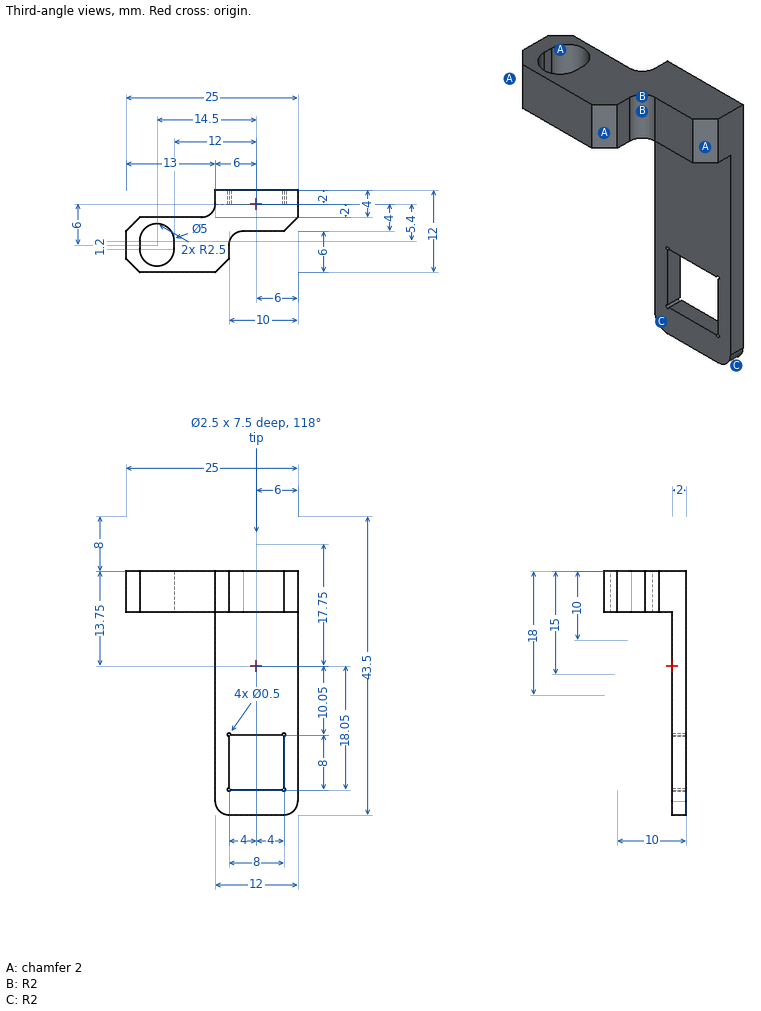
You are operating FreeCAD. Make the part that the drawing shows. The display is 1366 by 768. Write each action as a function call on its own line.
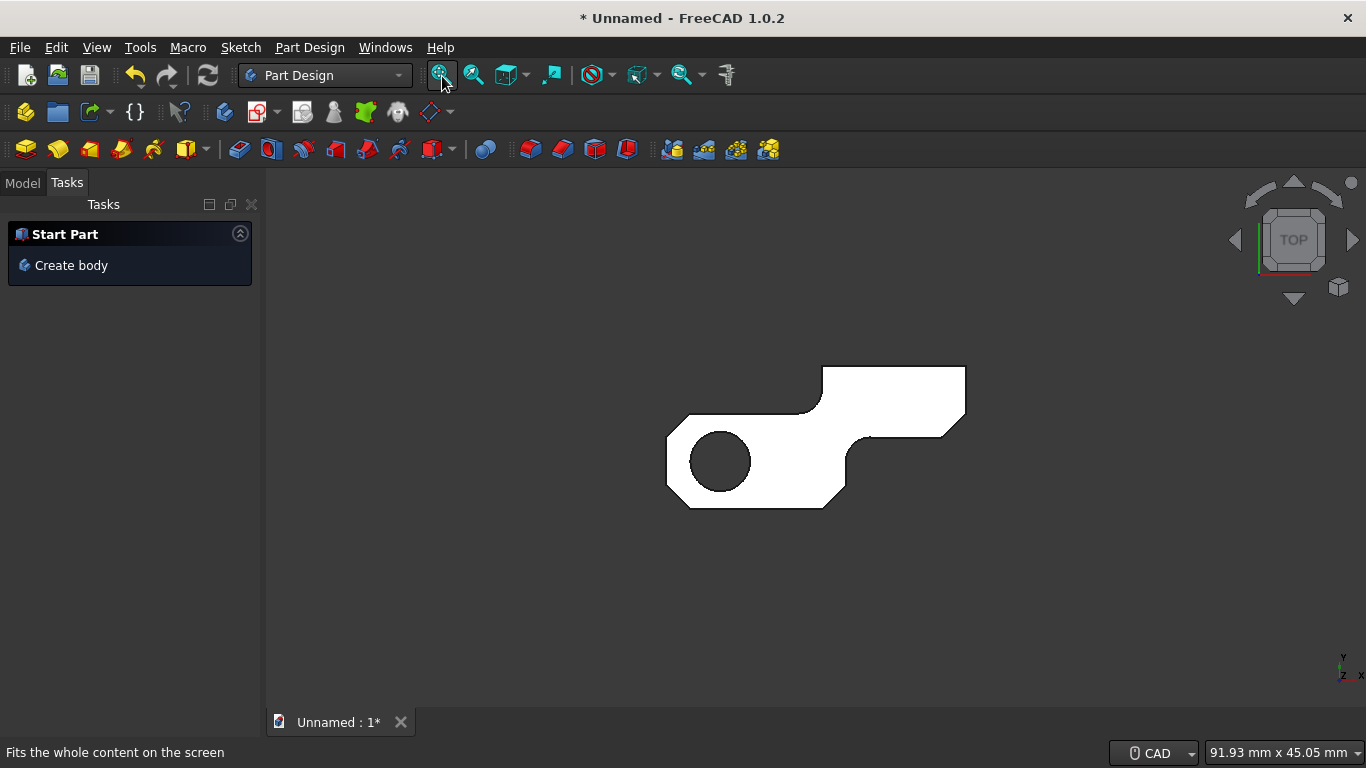
key(0)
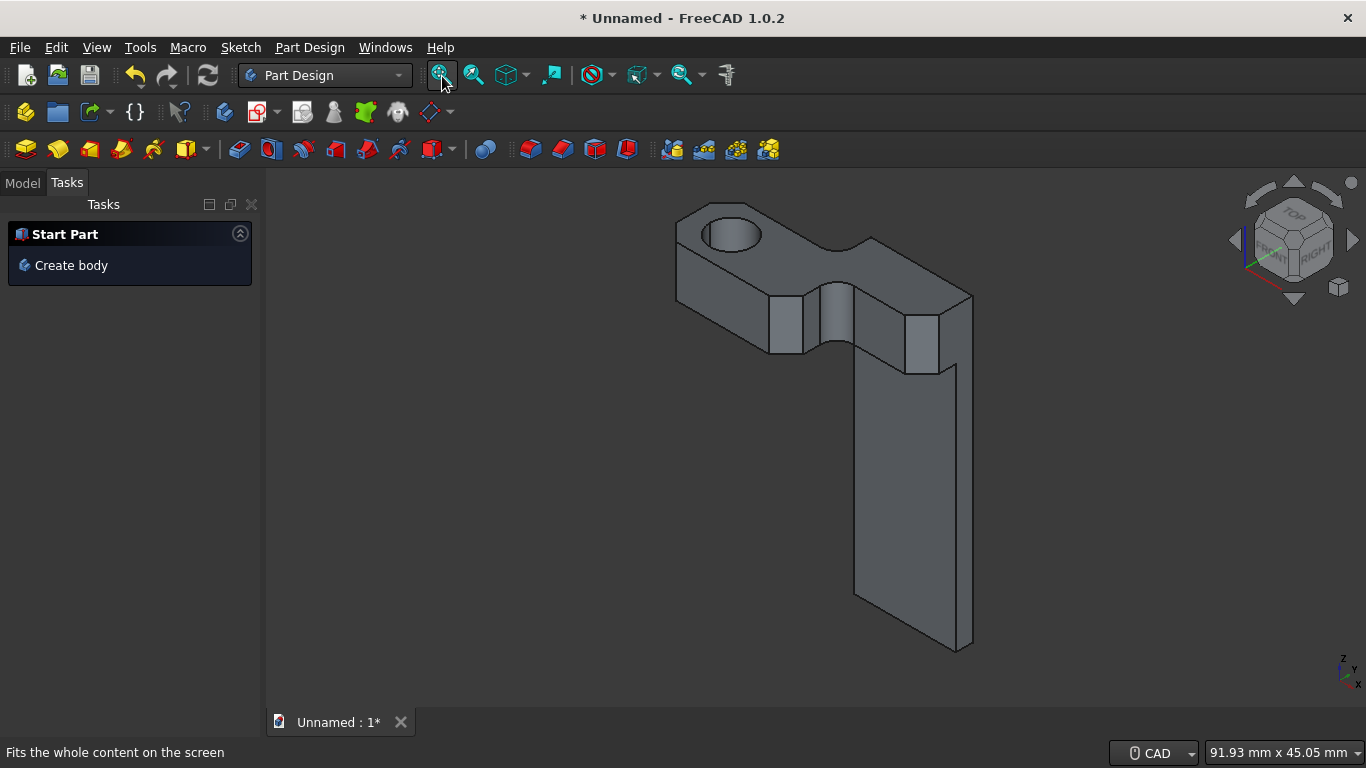
key(1)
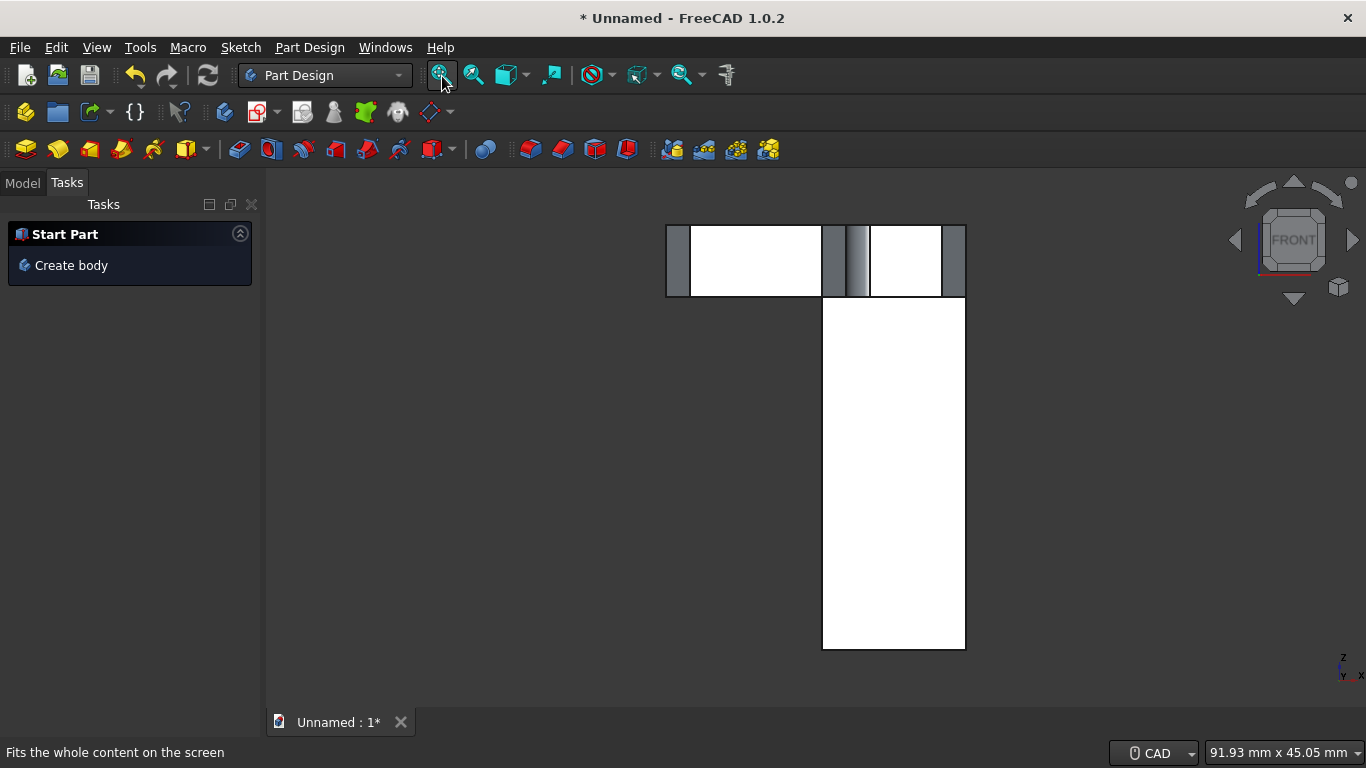
key(3)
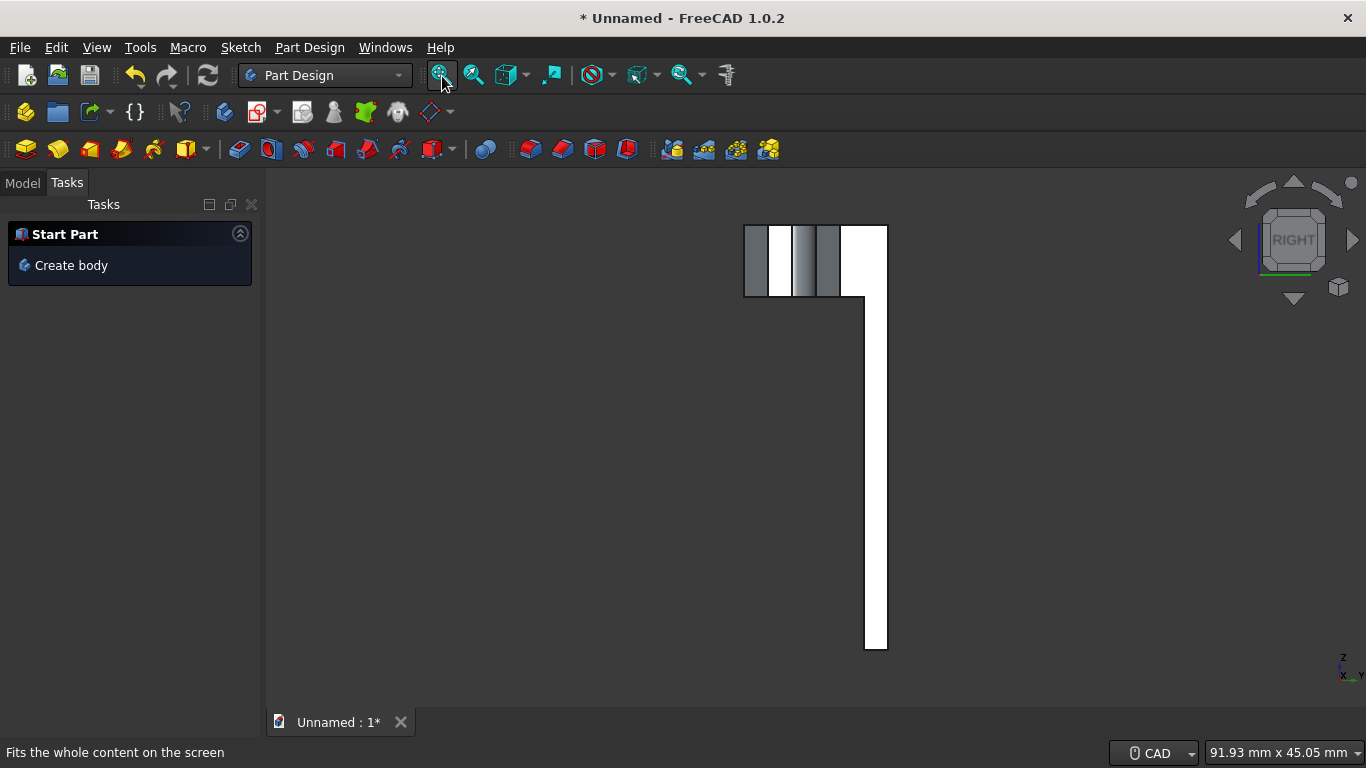
click(876, 649)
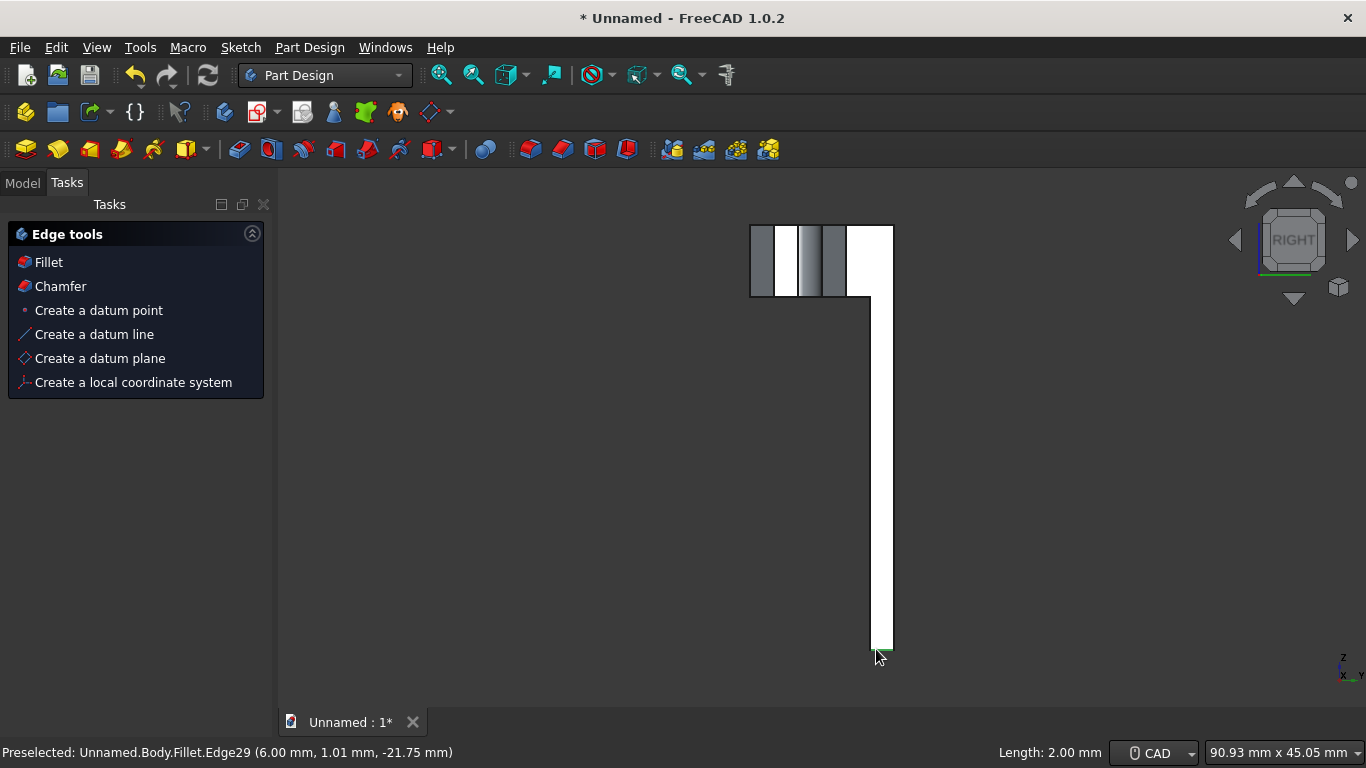
key(5)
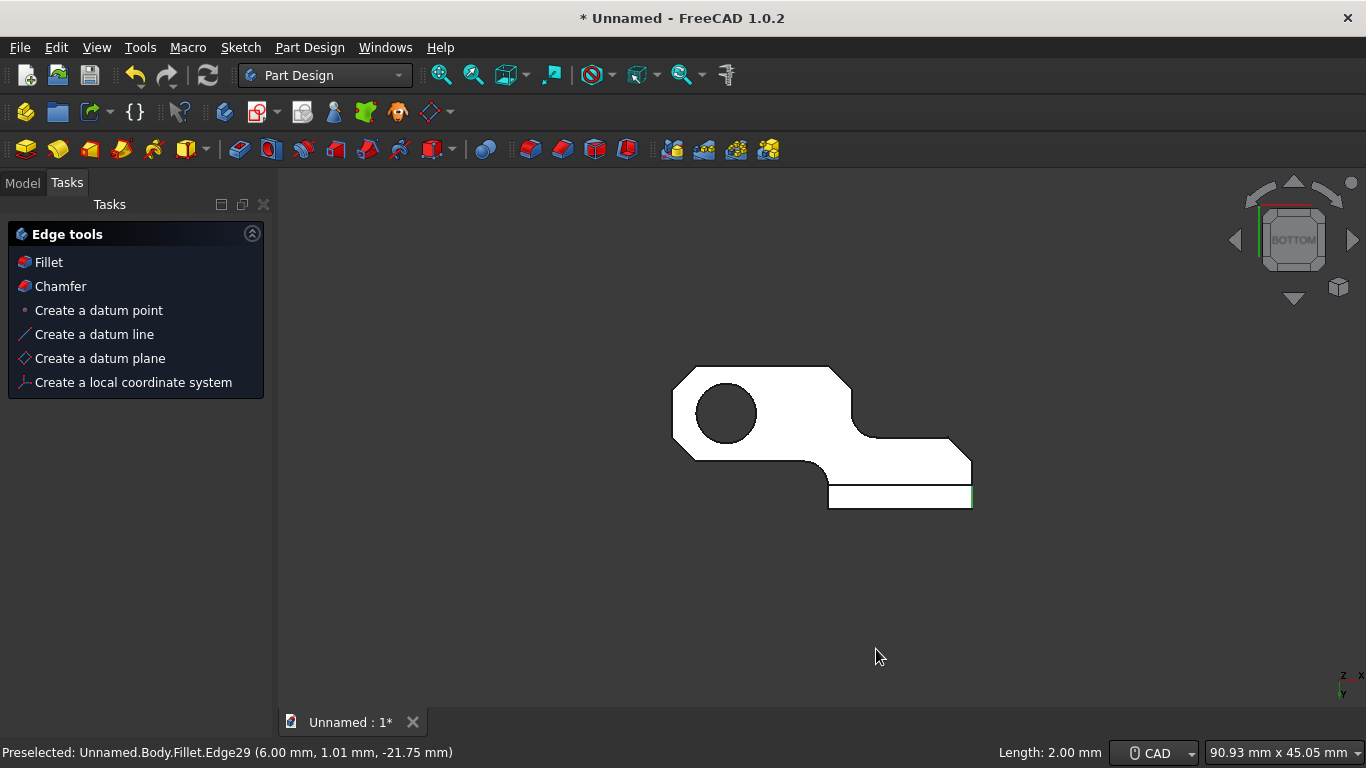
click(442, 76)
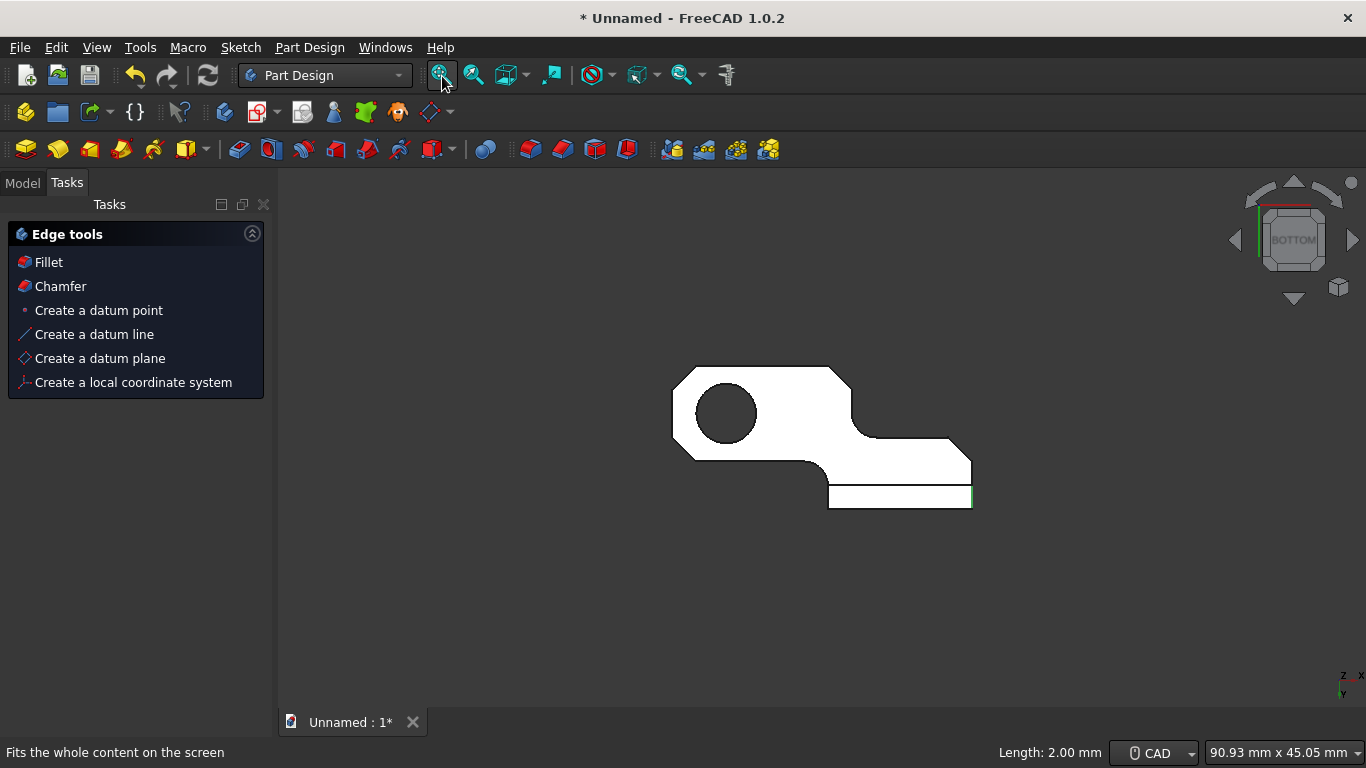
click(828, 496, ctrl)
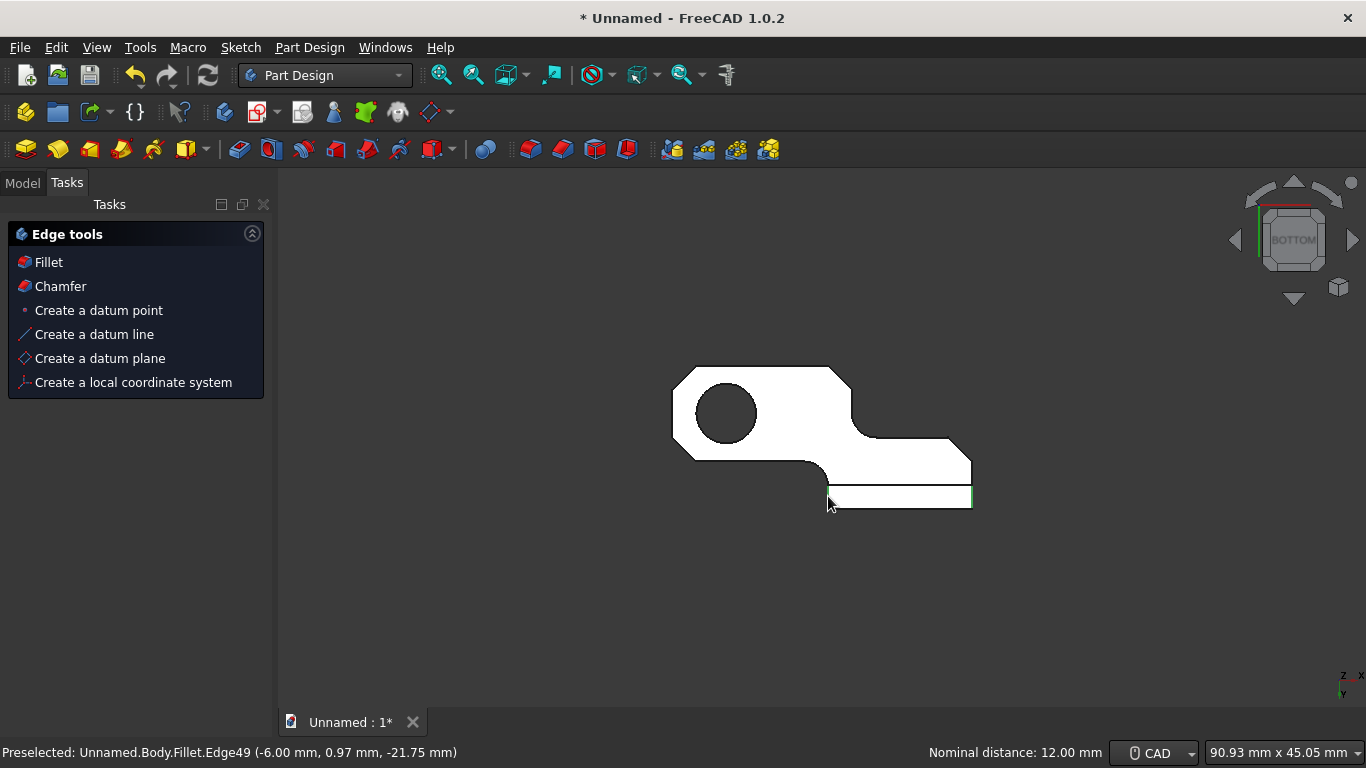
click(532, 150)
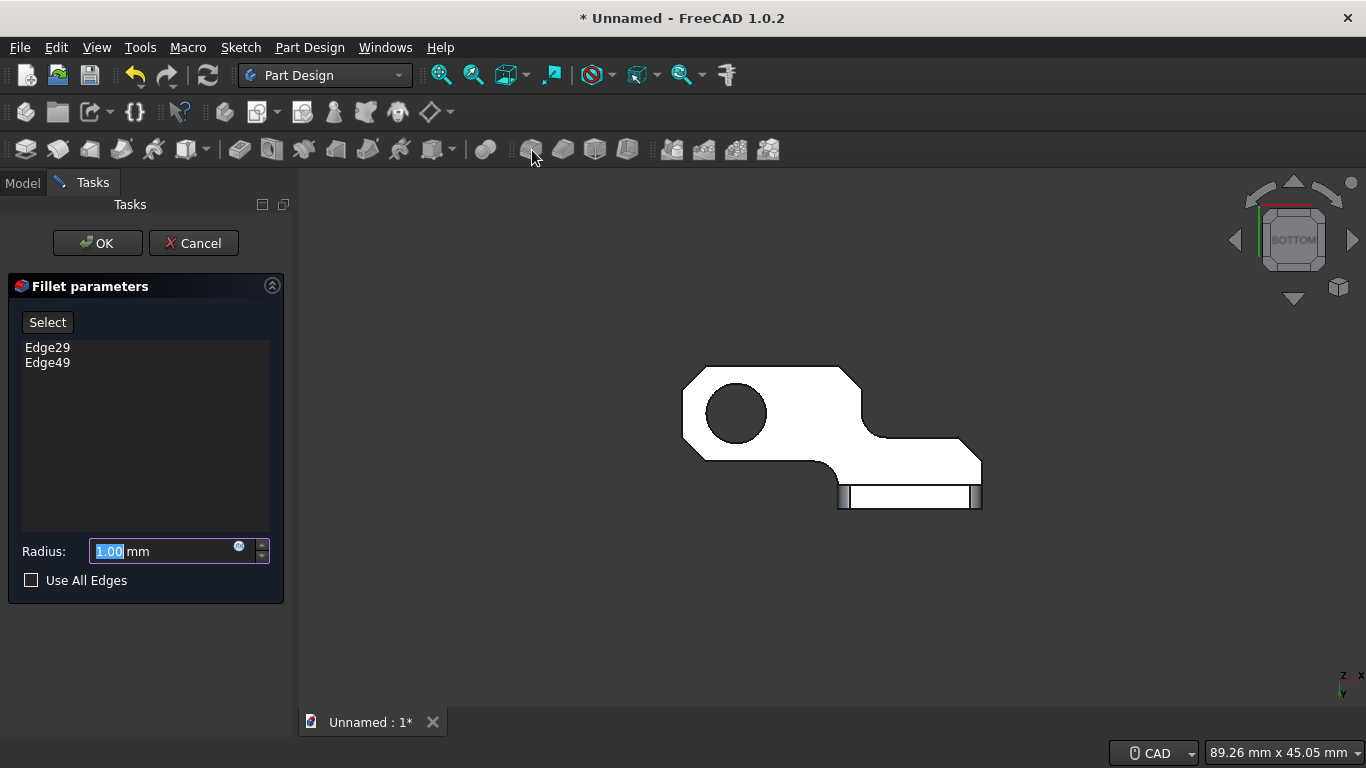
text(2)
key(Tab)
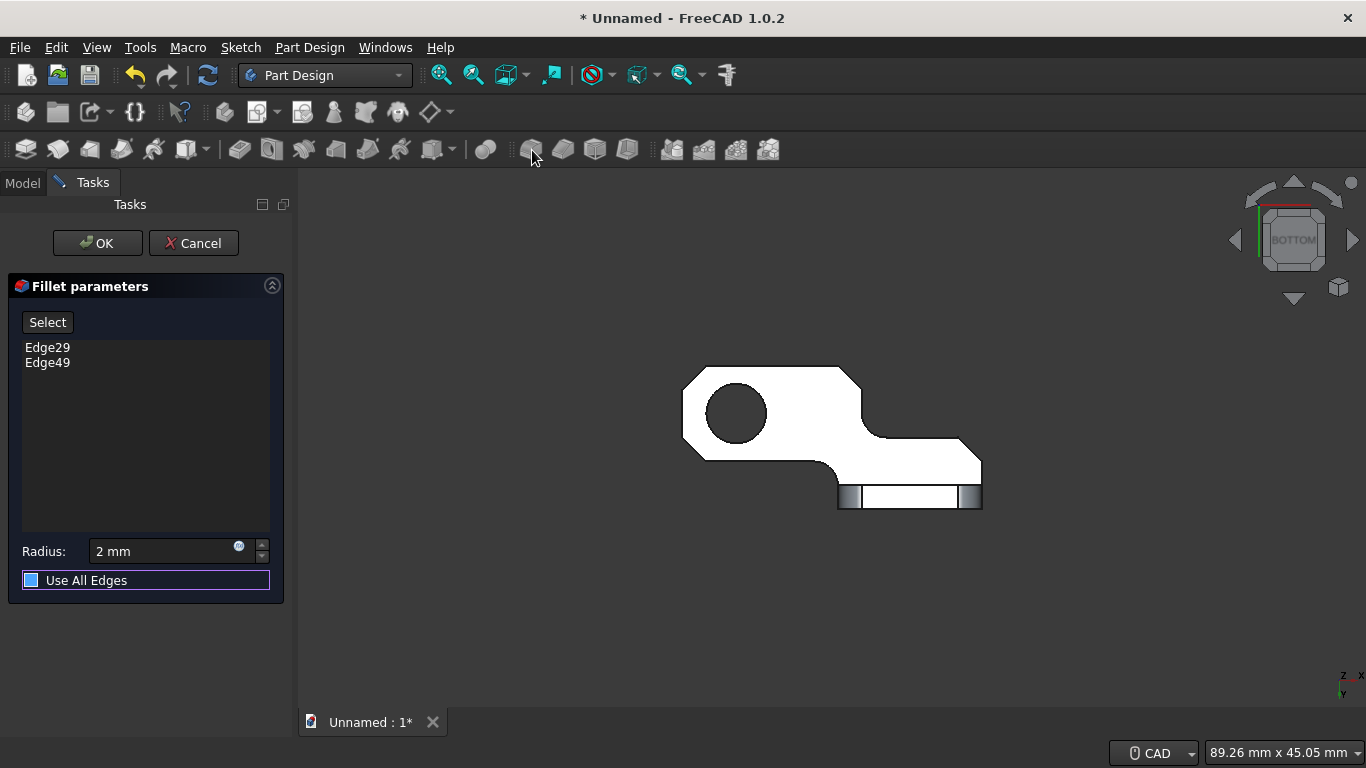
click(98, 243)